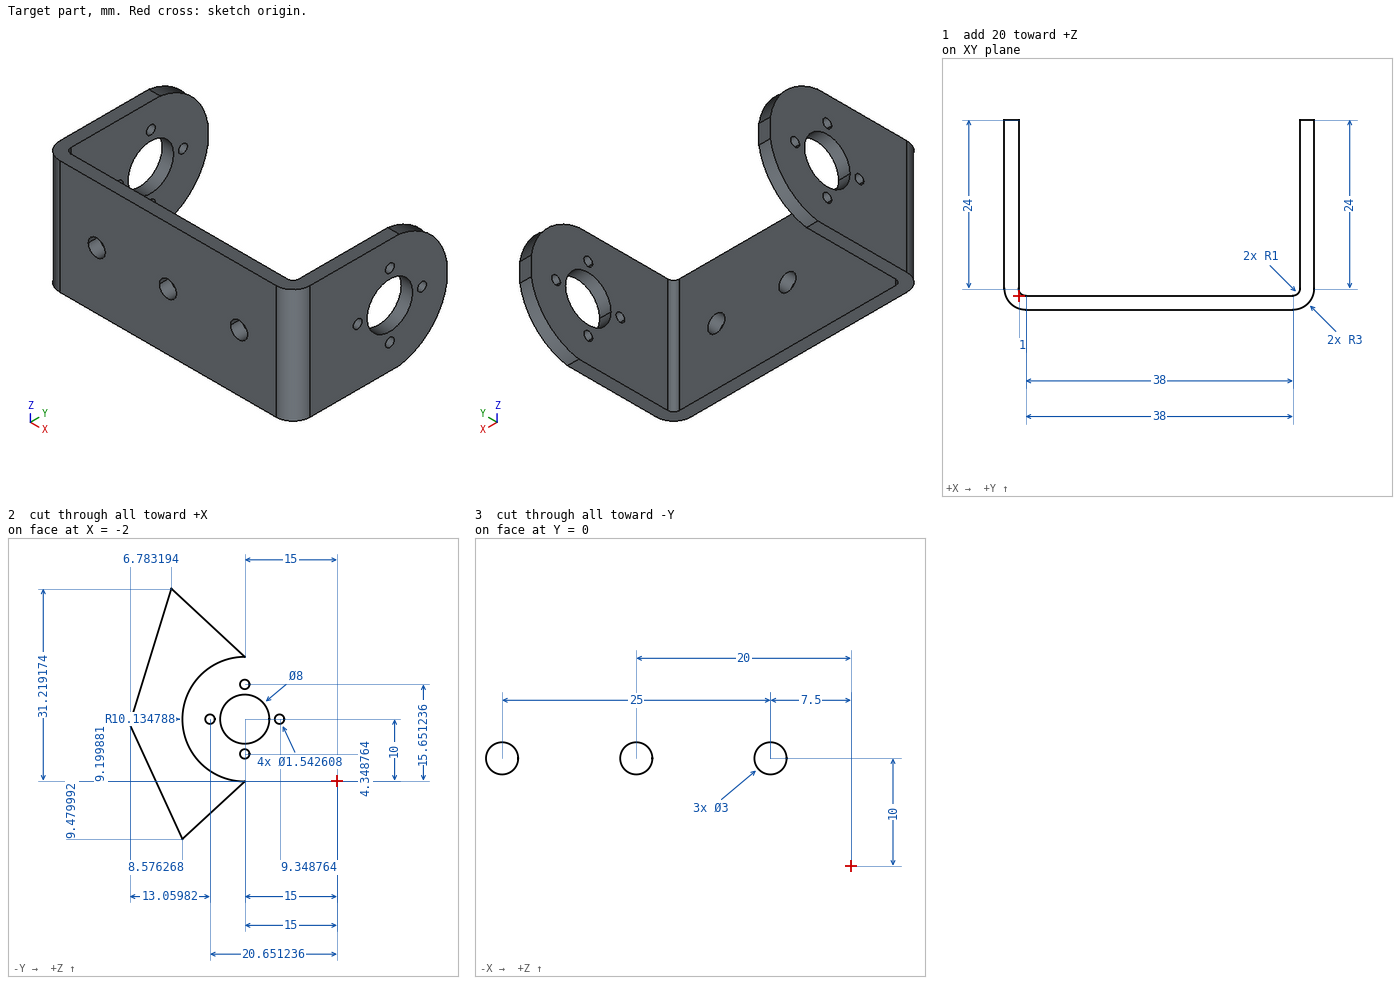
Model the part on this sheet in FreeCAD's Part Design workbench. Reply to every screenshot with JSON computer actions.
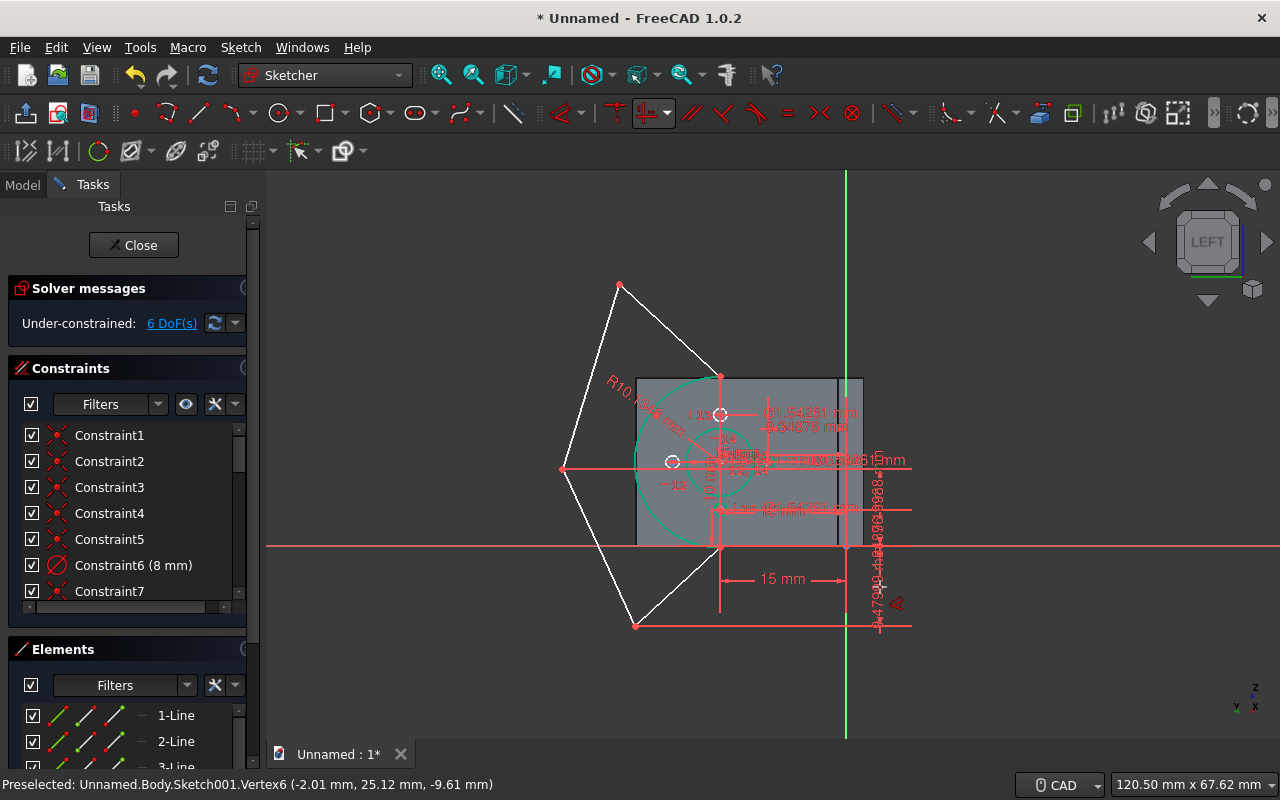
{"action": "left_click", "coordinate": [603, 340]}
{"action": "left_click", "coordinate": [591, 250]}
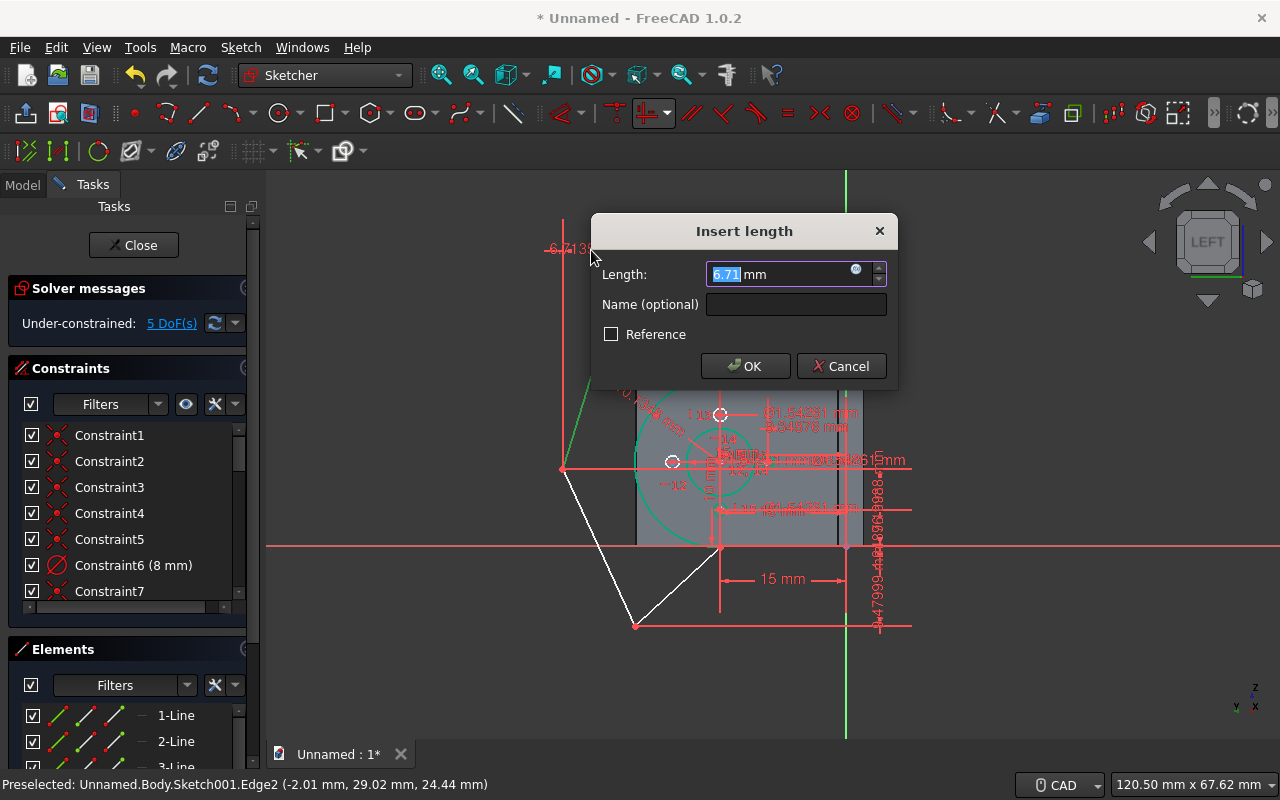
{"action": "type", "text": "6.783194"}
{"action": "key", "text": "Return"}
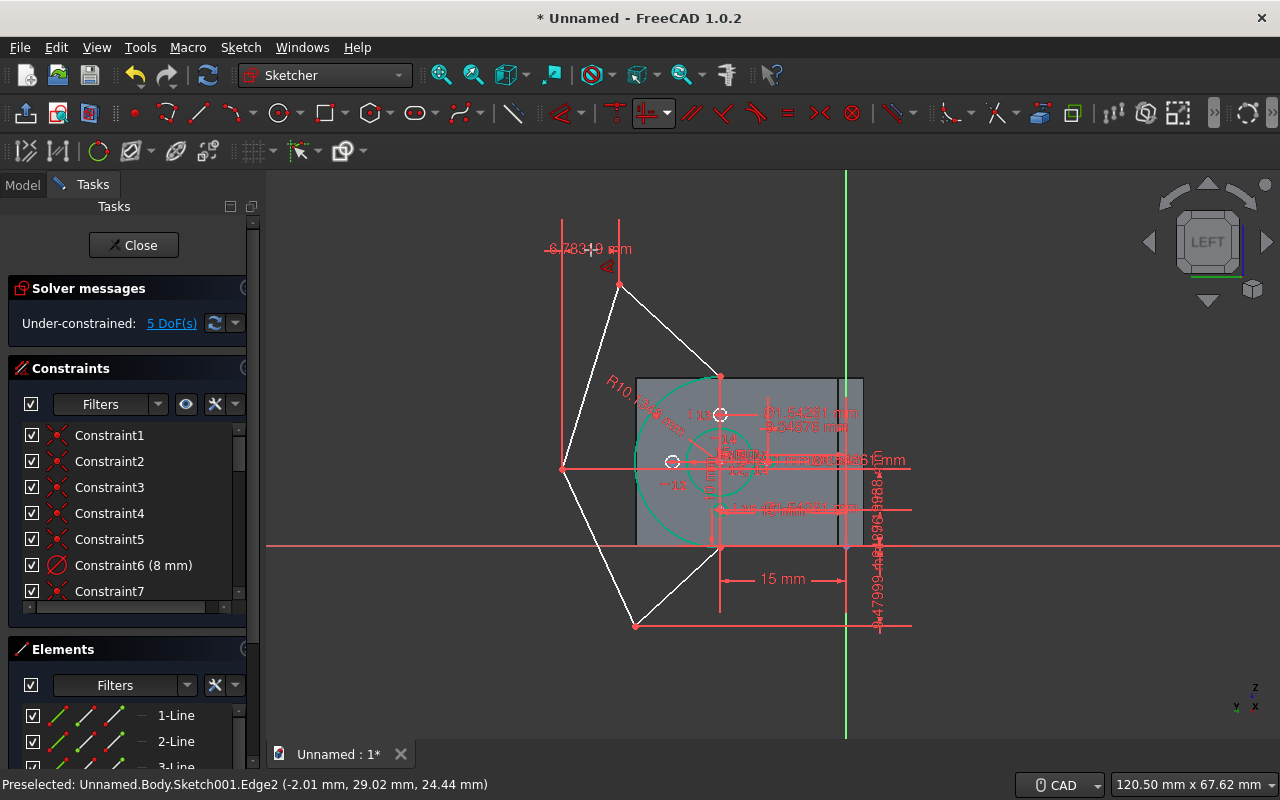
{"action": "left_click", "coordinate": [584, 516]}
{"action": "left_click", "coordinate": [599, 660]}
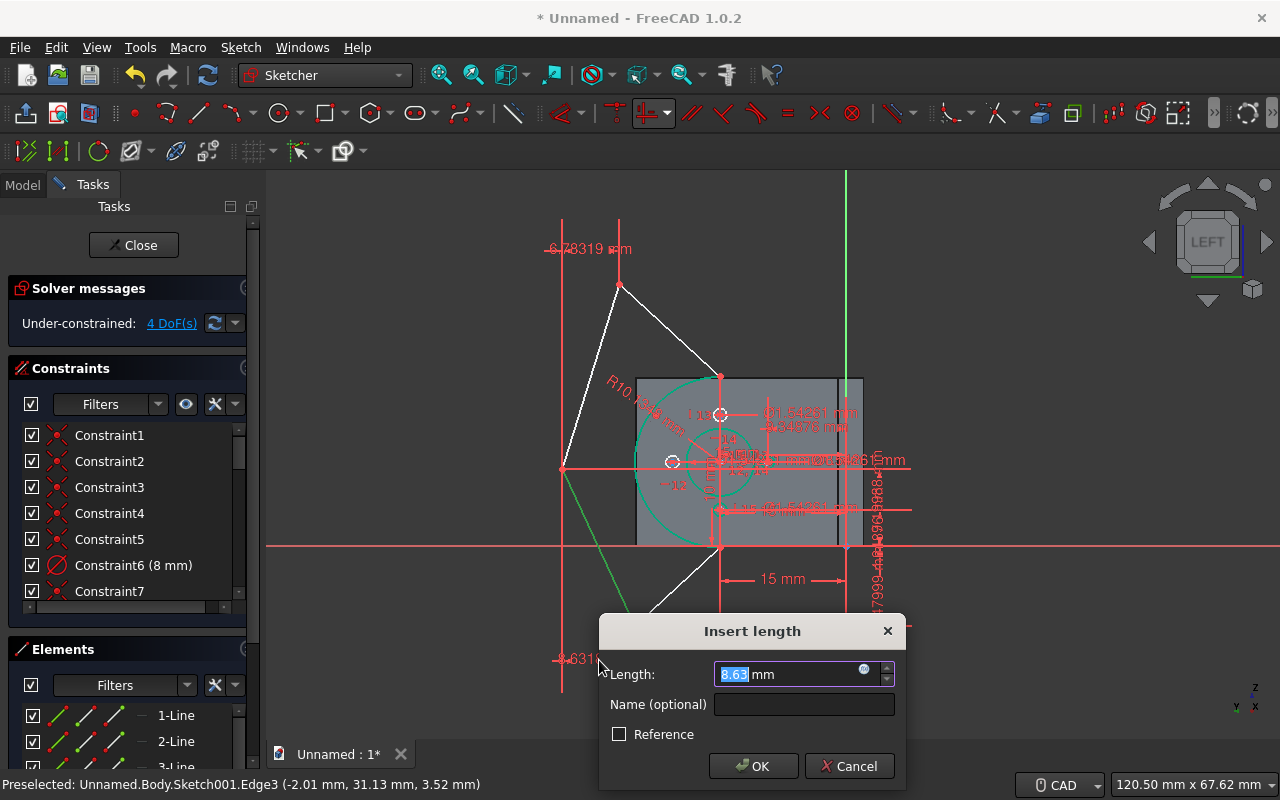
{"action": "type", "text": "8.576268"}
{"action": "key", "text": "Return"}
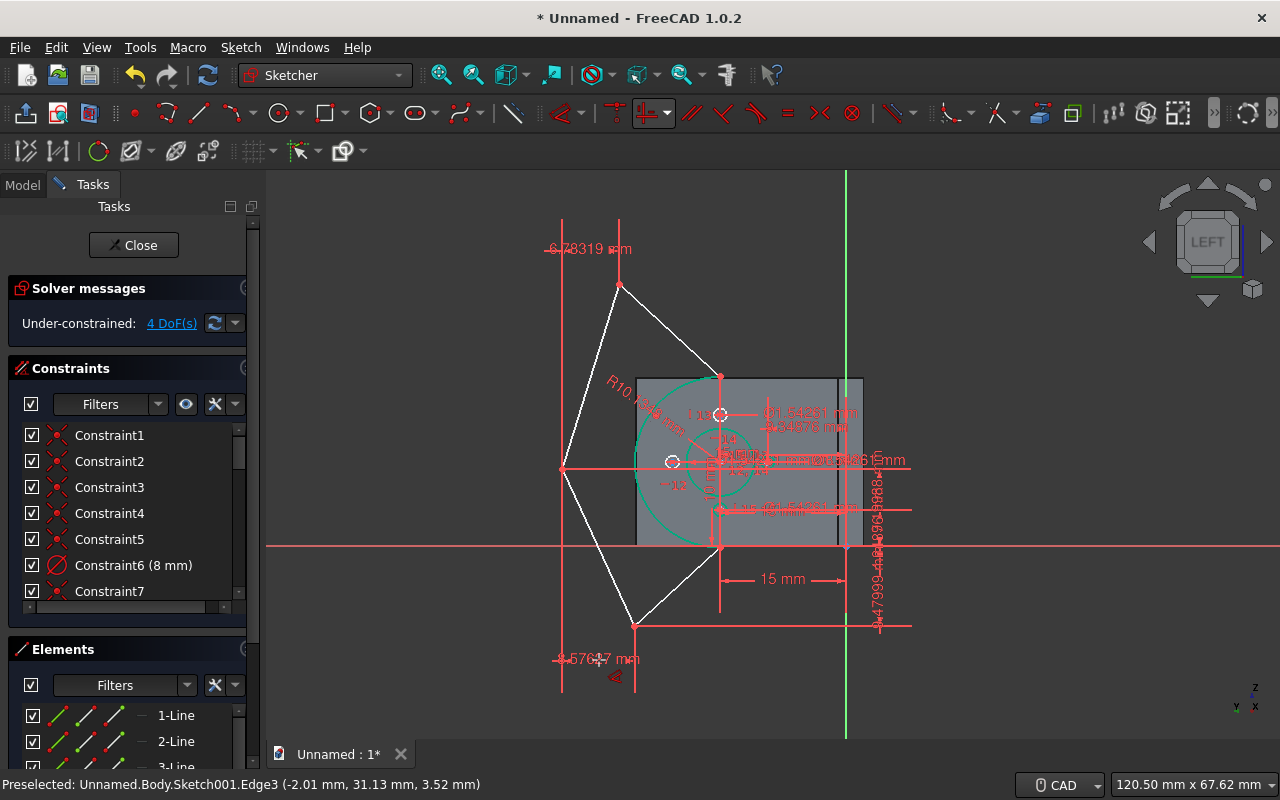
{"action": "left_click", "coordinate": [673, 462]}
{"action": "left_click", "coordinate": [759, 604]}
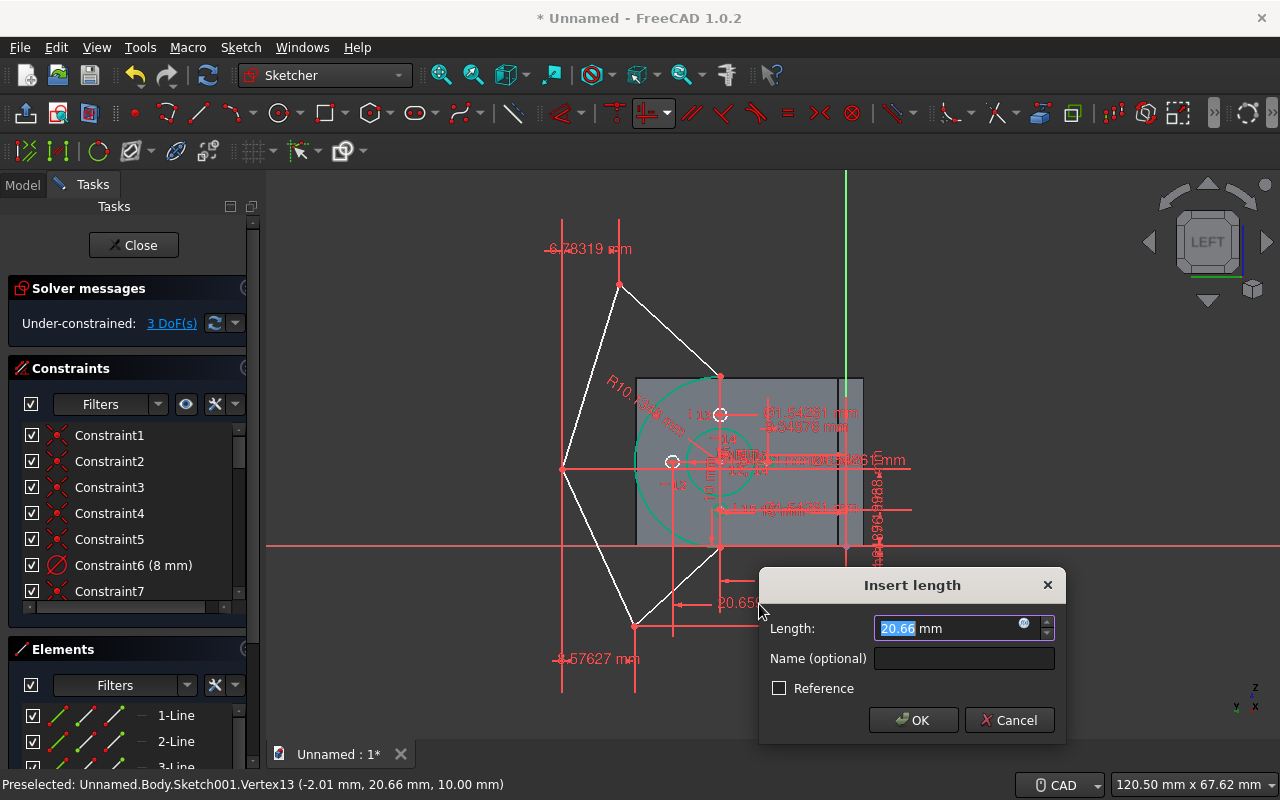
{"action": "type", "text": "20.651236"}
{"action": "key", "text": "Return"}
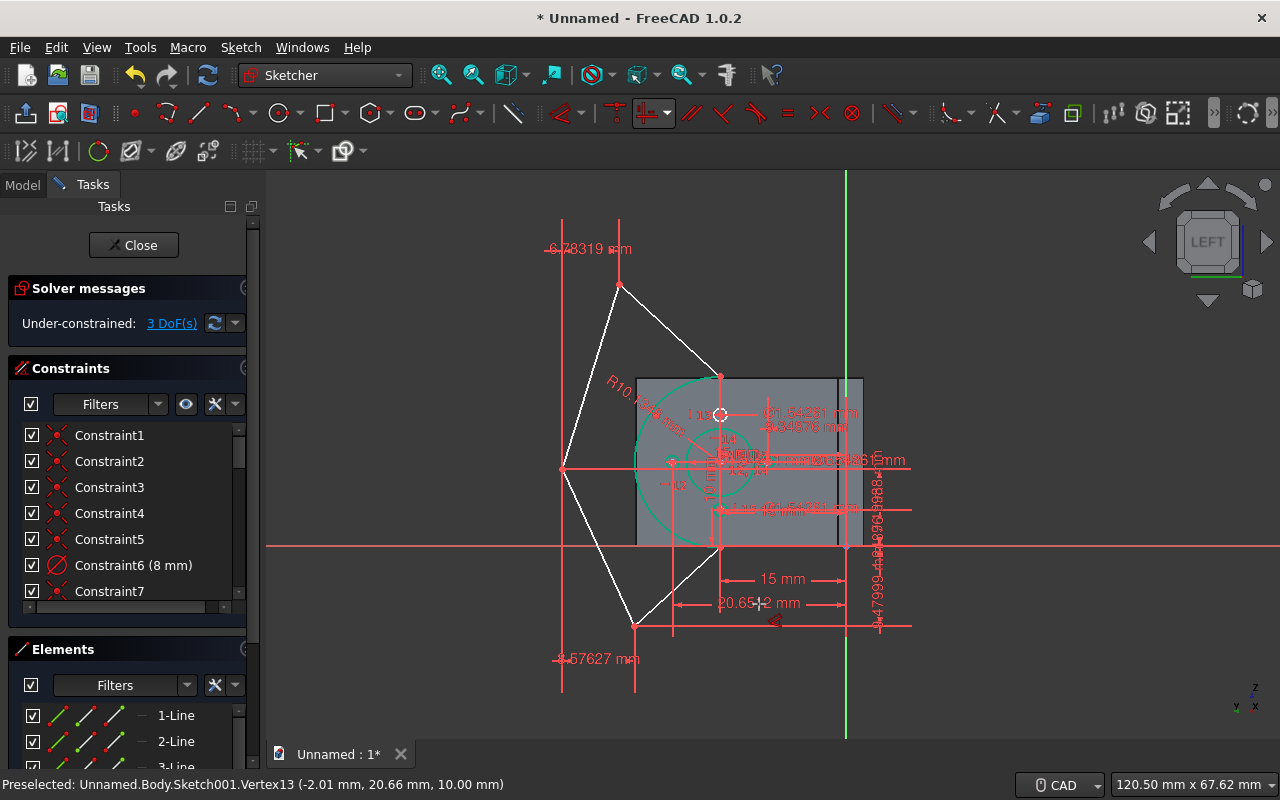
{"action": "left_click", "coordinate": [720, 415]}
{"action": "left_click", "coordinate": [880, 451]}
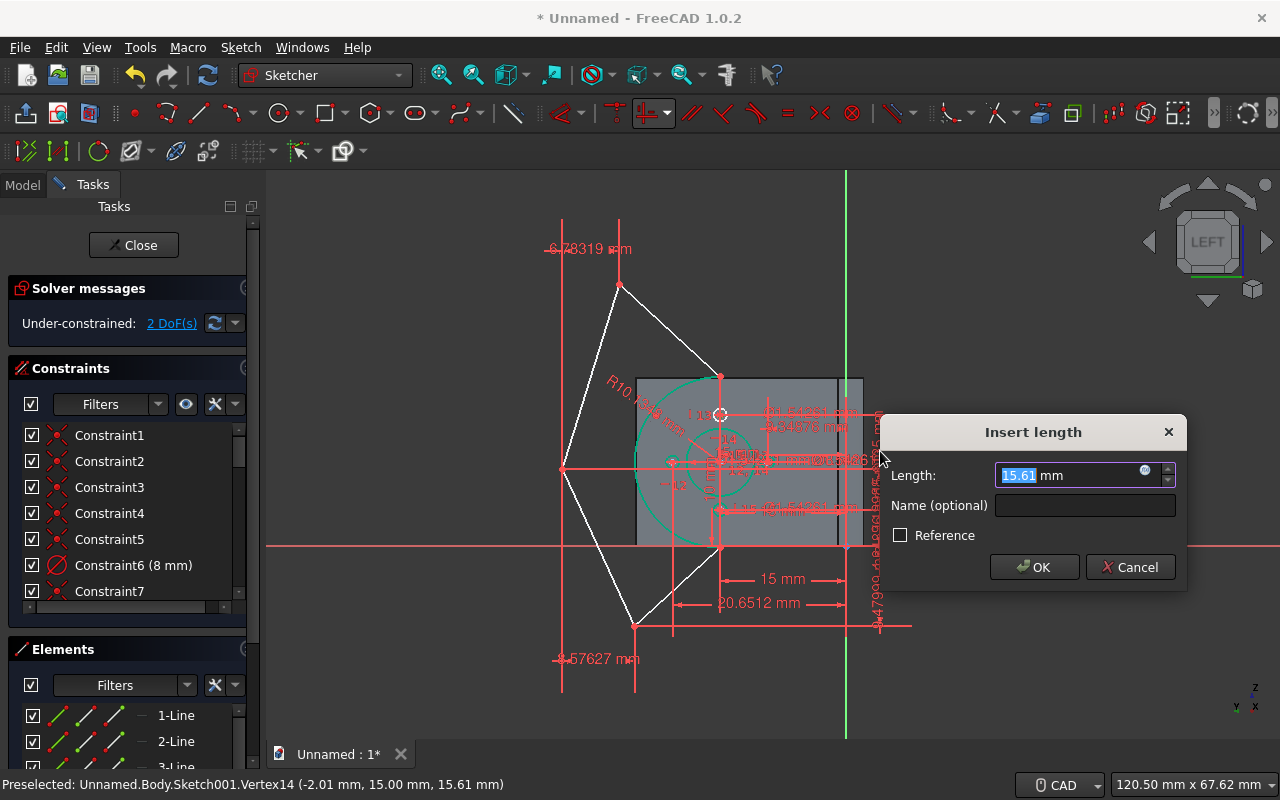
{"action": "type", "text": "15.651236"}
{"action": "key", "text": "Return"}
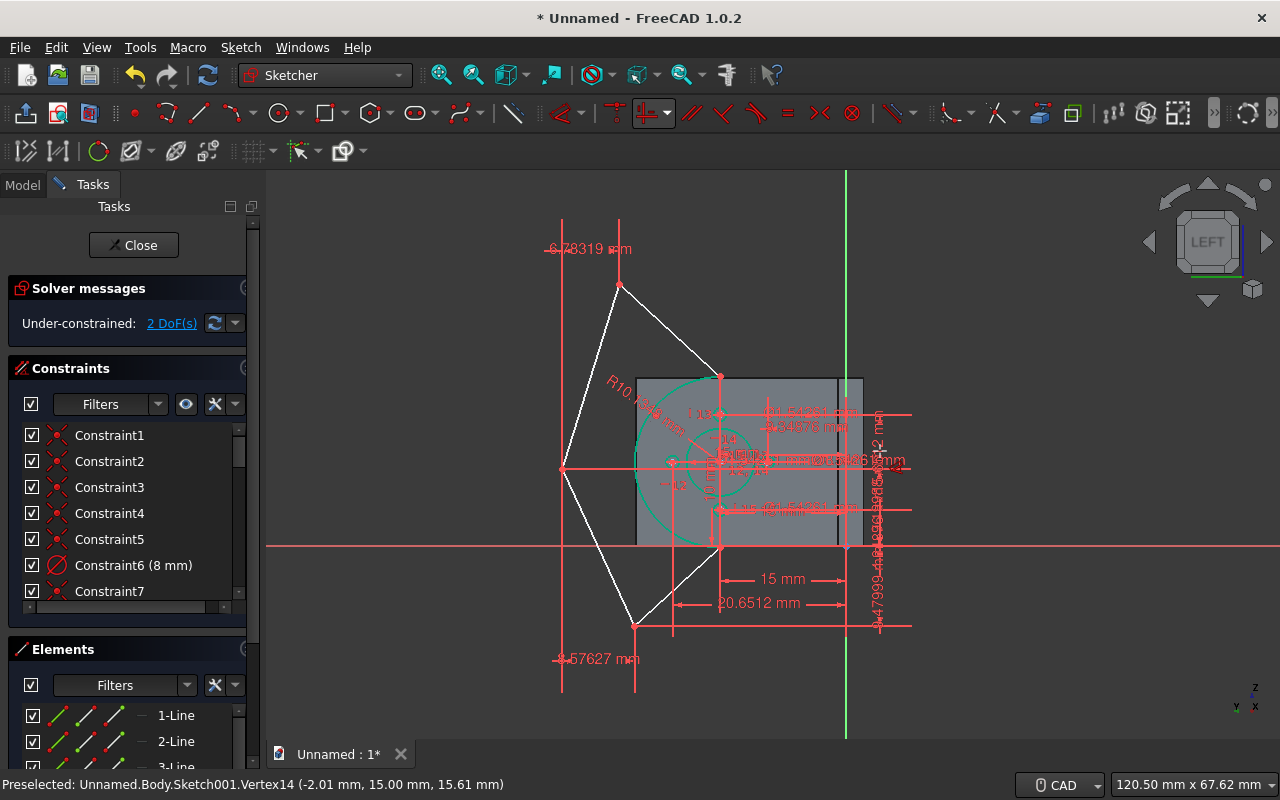
{"action": "left_click", "coordinate": [562, 469]}